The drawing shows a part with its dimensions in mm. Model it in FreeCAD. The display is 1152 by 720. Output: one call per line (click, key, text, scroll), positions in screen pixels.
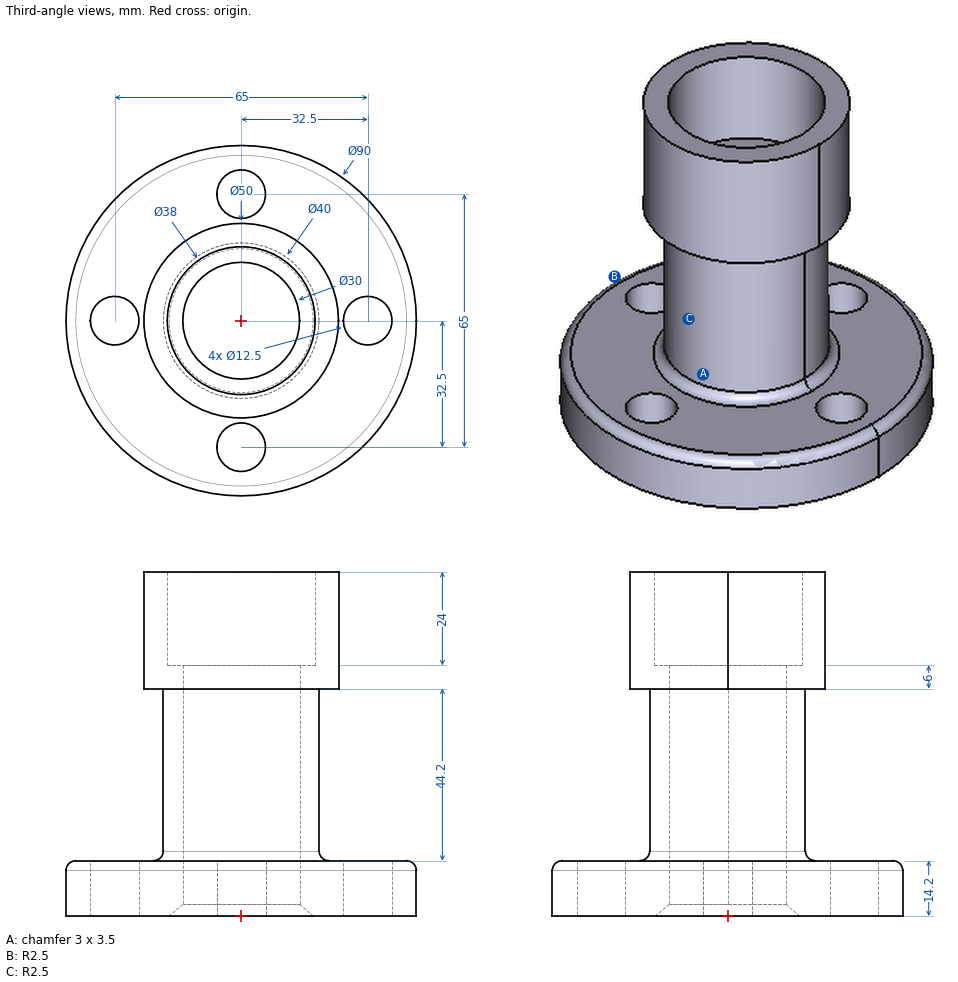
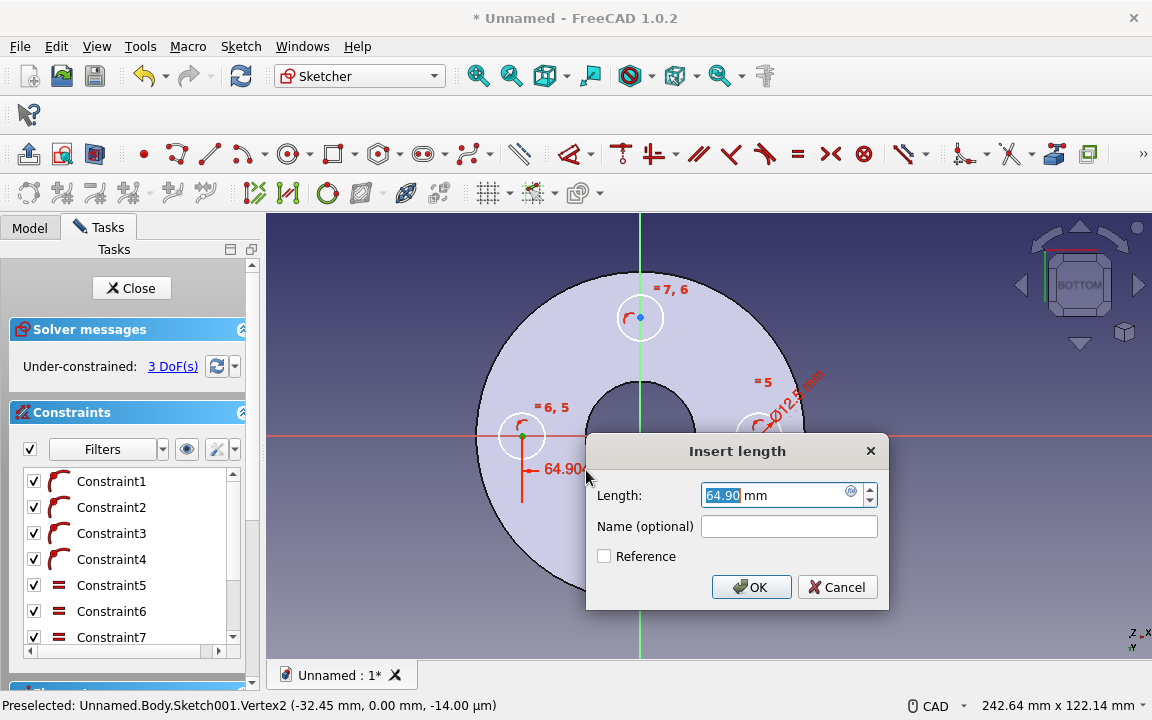
text(65)
key(Return)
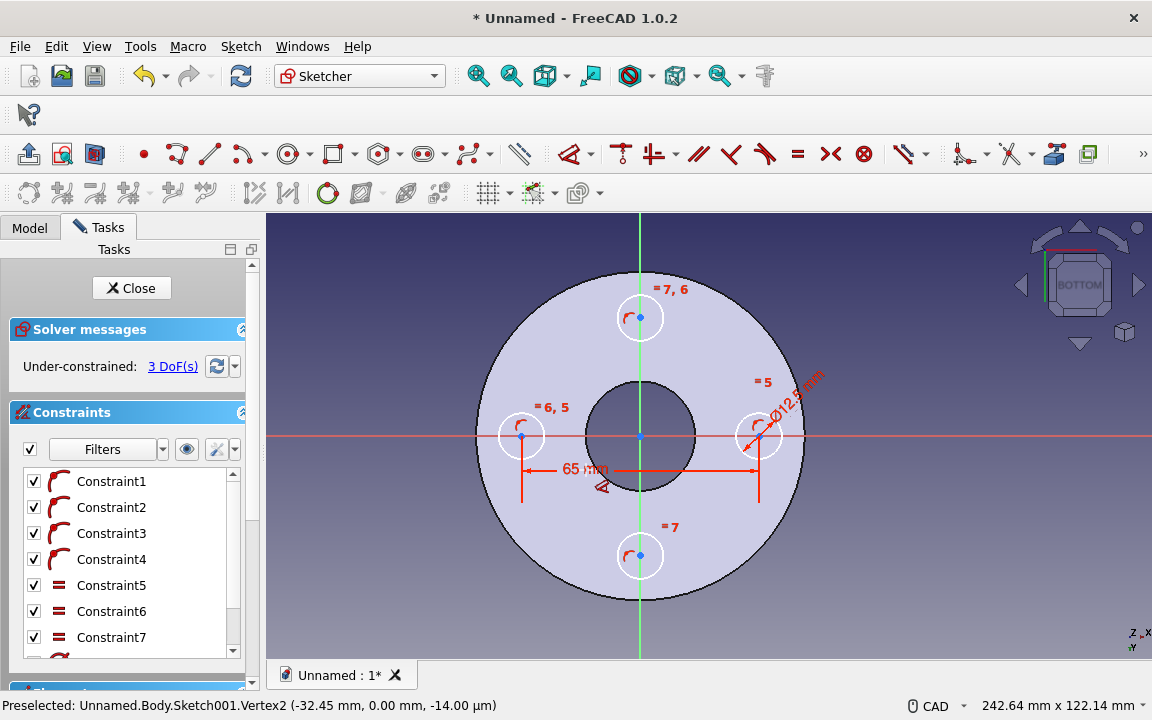
click(640, 318)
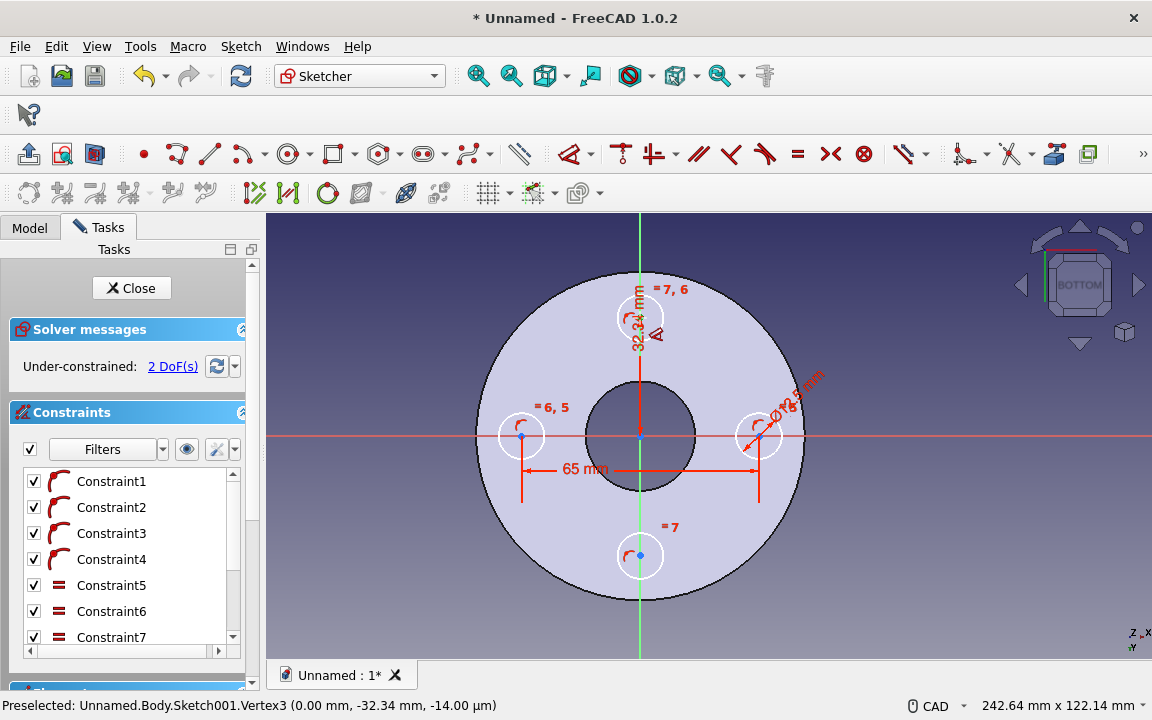
click(640, 556)
click(674, 382)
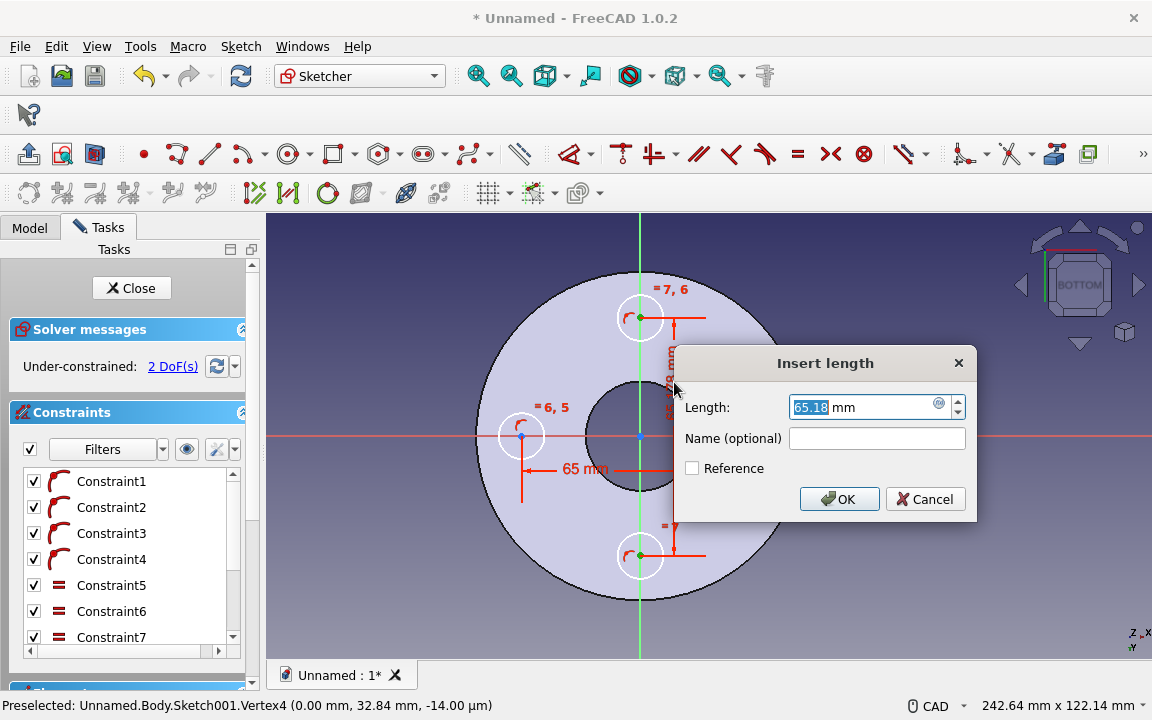
text(65)
key(Return)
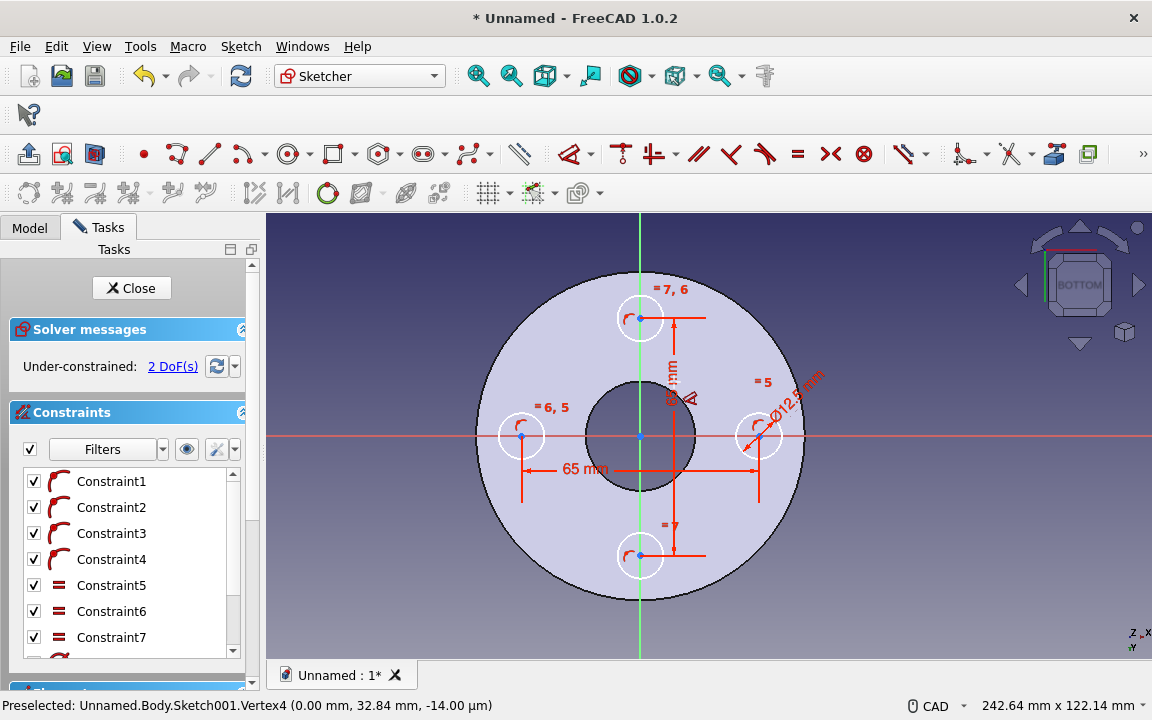
click(759, 436)
click(700, 470)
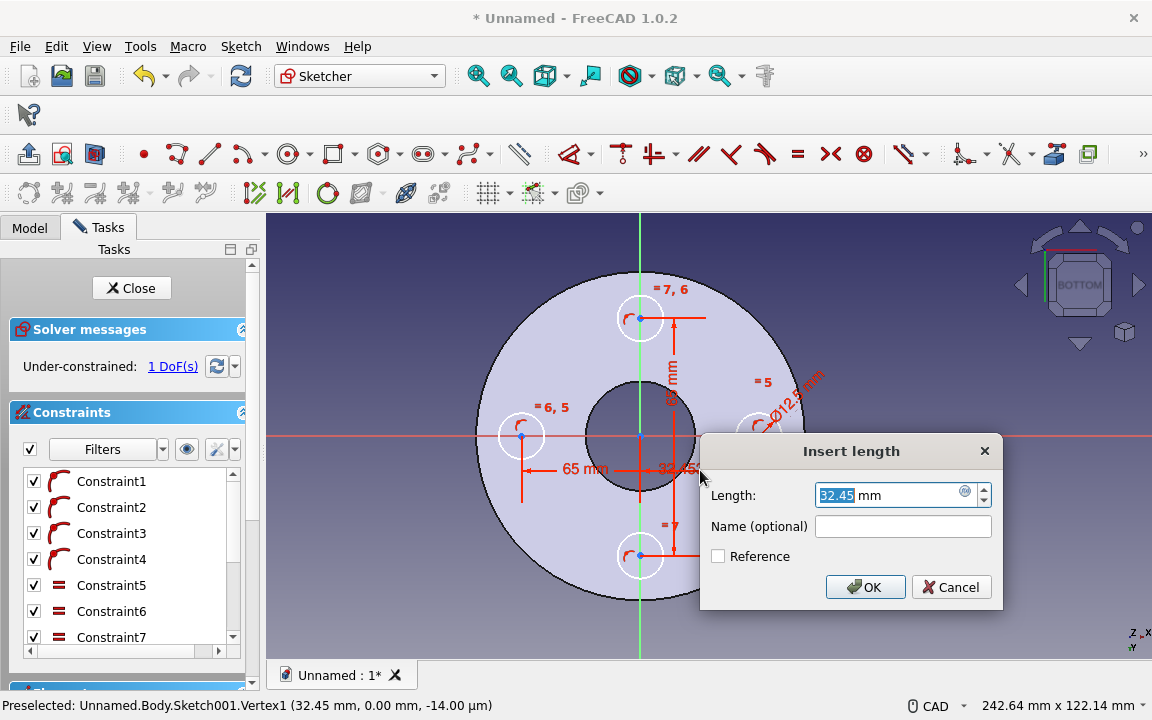
text(32.5)
key(Return)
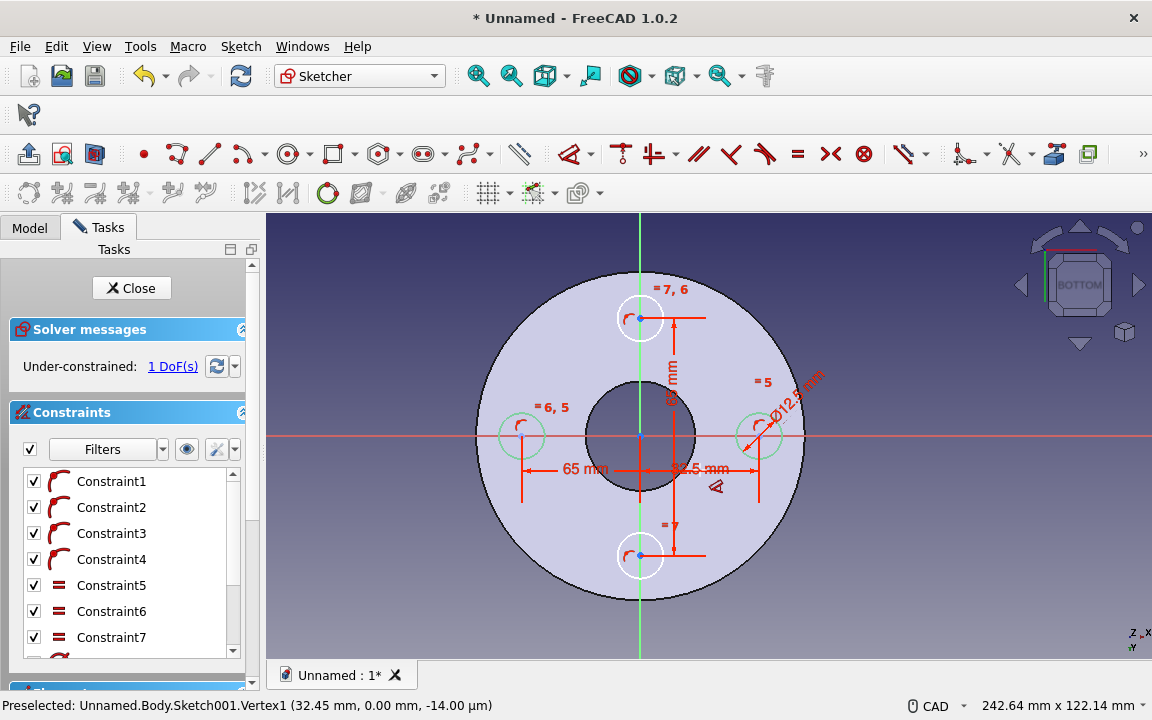
click(640, 318)
click(674, 350)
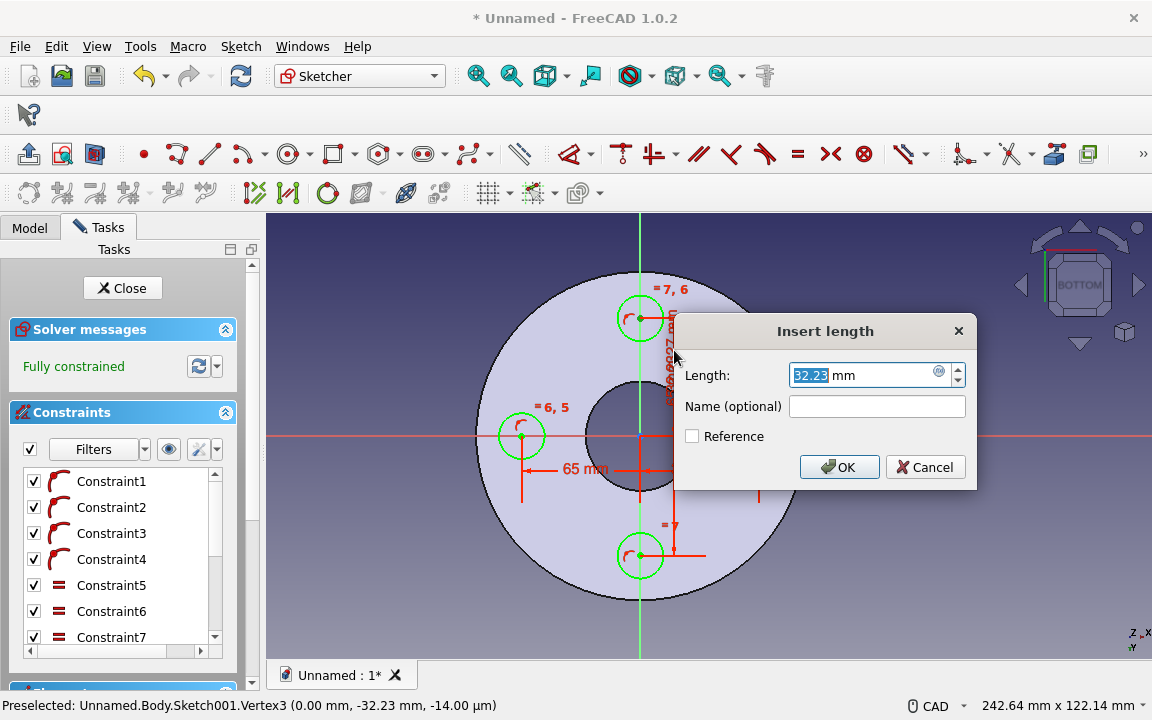
text(32.5)
key(Return)
key(Escape)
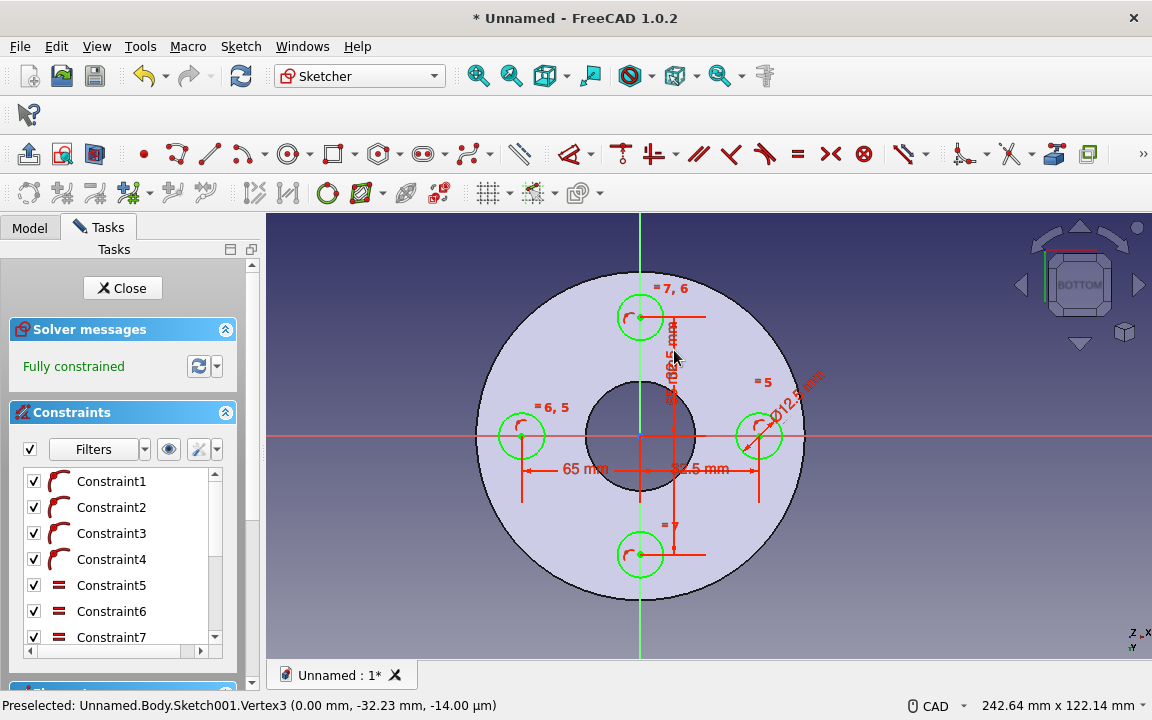
click(123, 288)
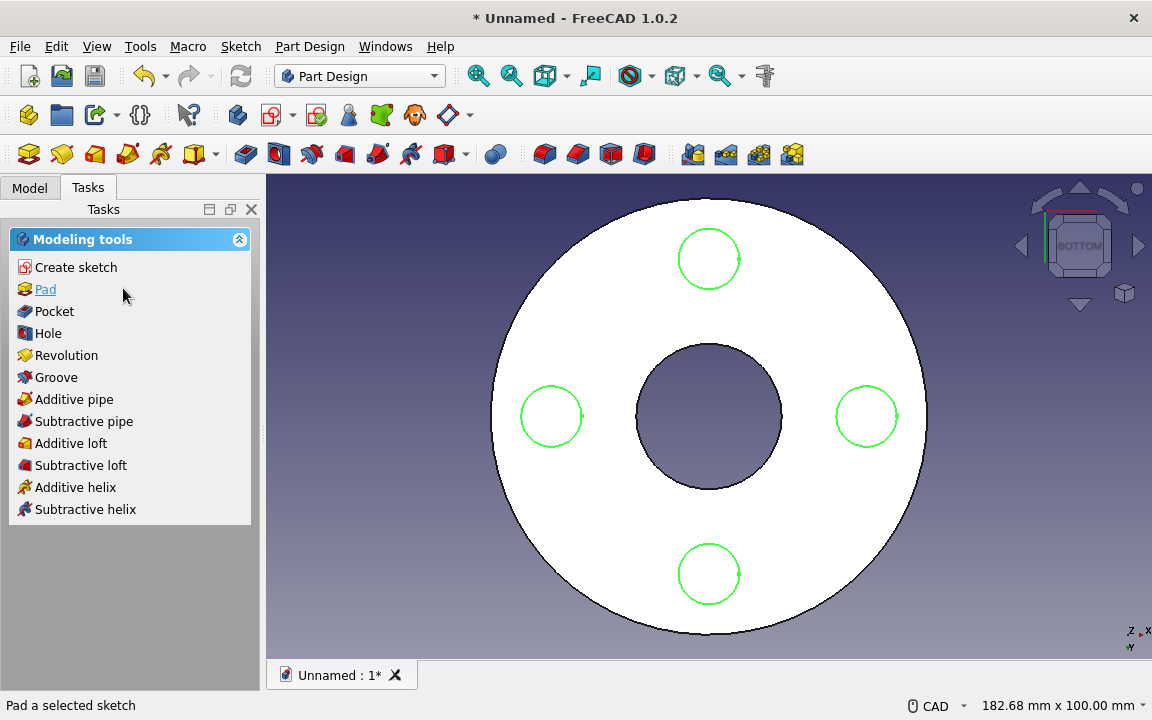
click(246, 154)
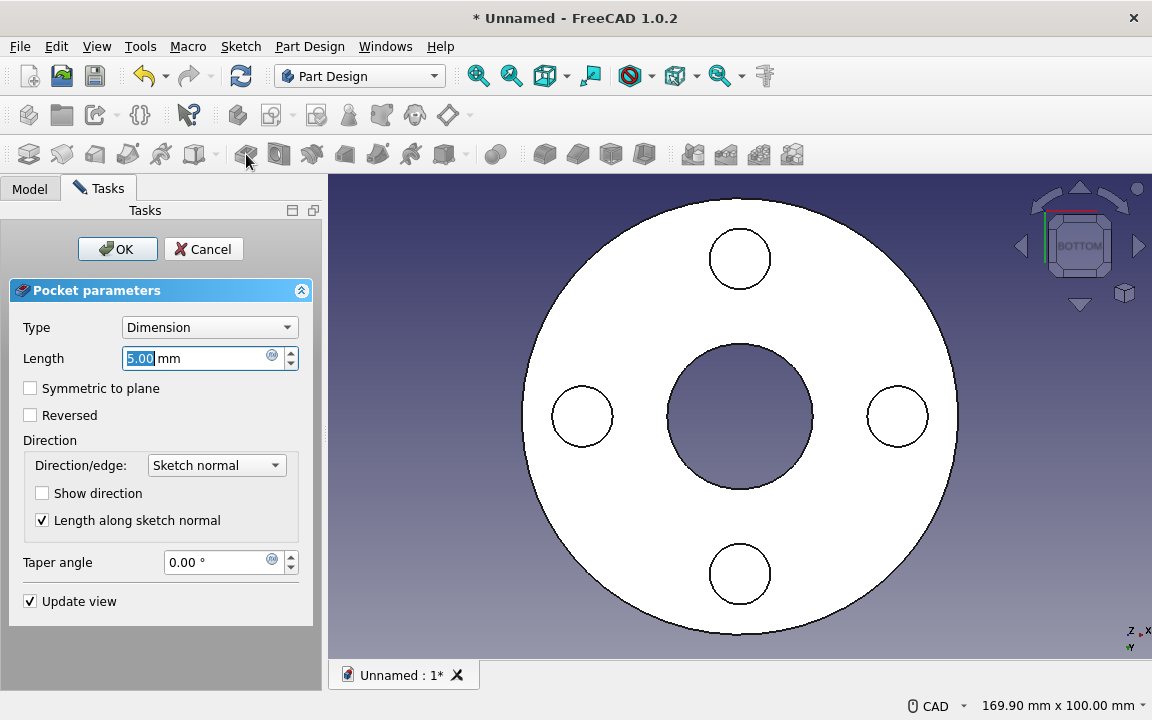
click(210, 328)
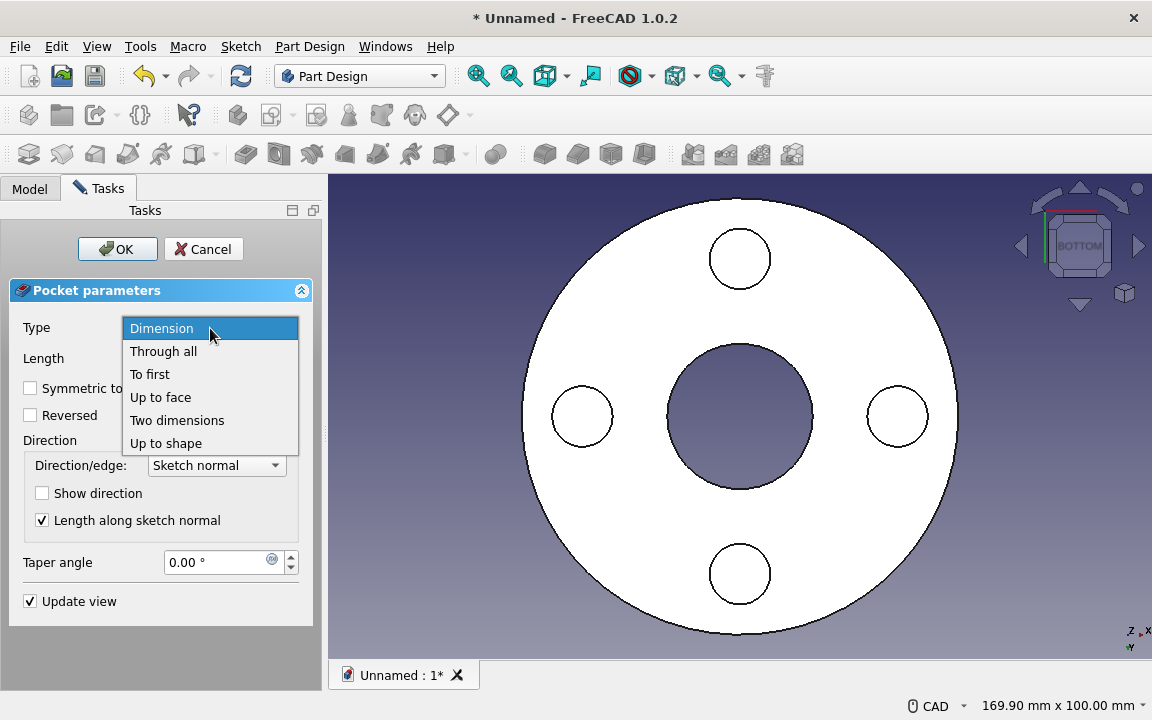
click(208, 352)